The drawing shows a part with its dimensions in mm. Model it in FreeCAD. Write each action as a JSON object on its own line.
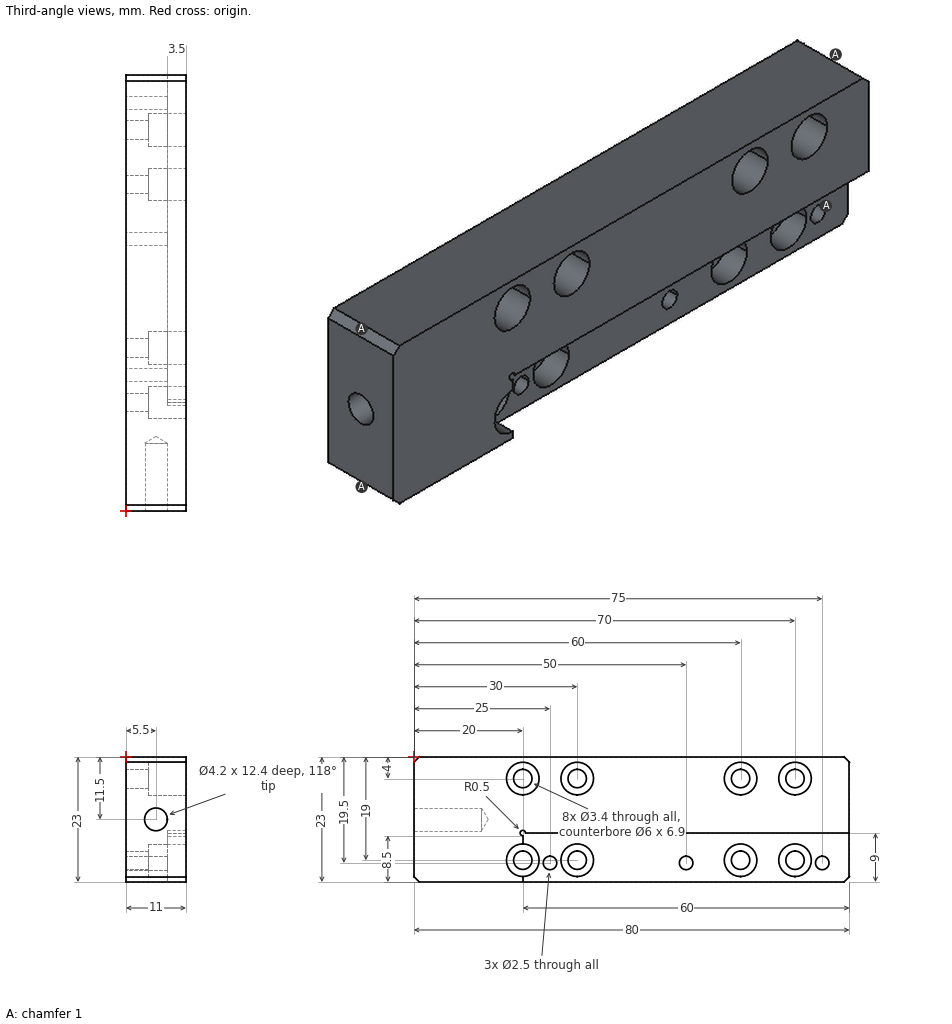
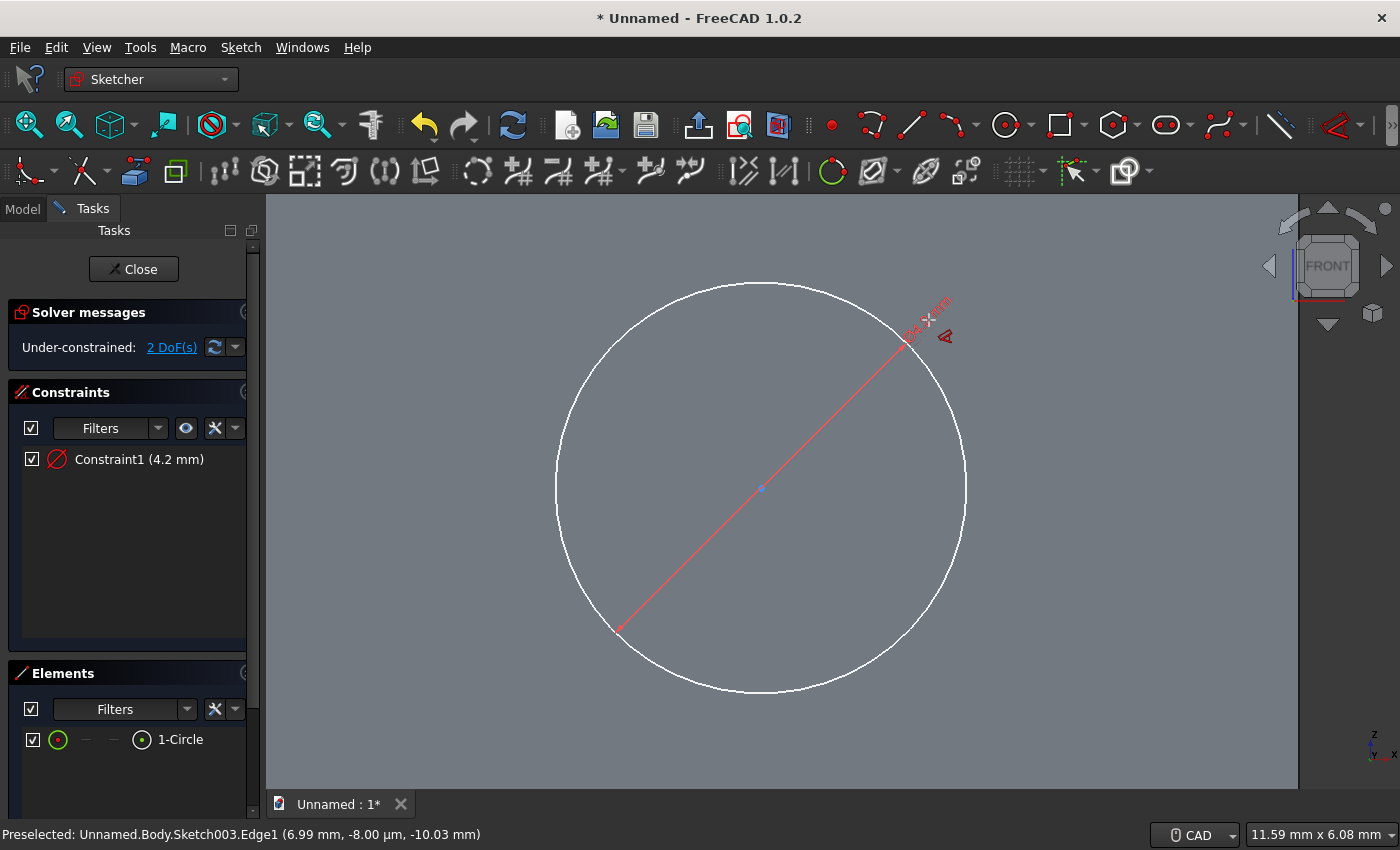
{"action": "left_click", "coordinate": [761, 488]}
{"action": "left_click", "coordinate": [528, 522]}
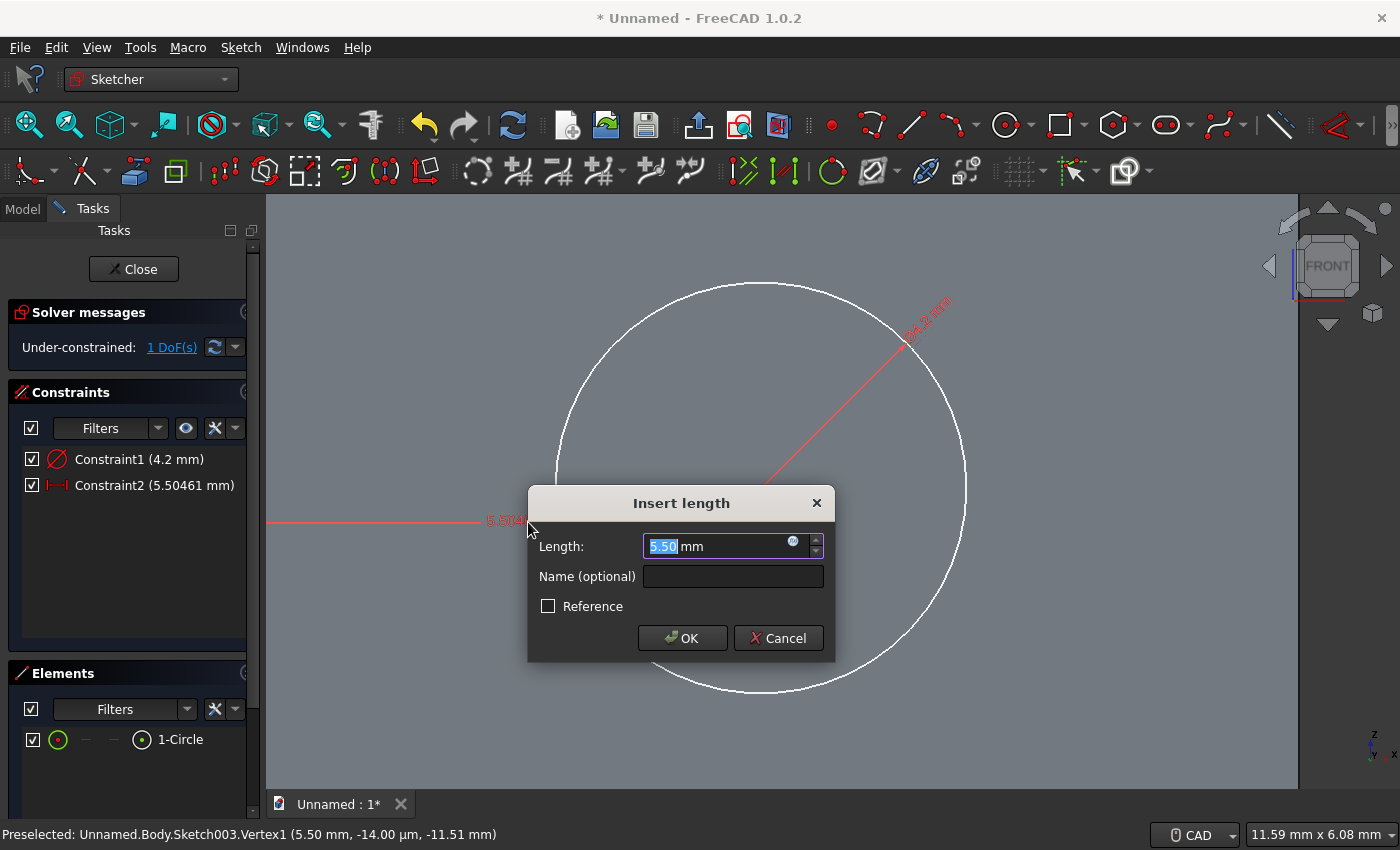
{"action": "type", "text": "5.5"}
{"action": "key", "text": "Return"}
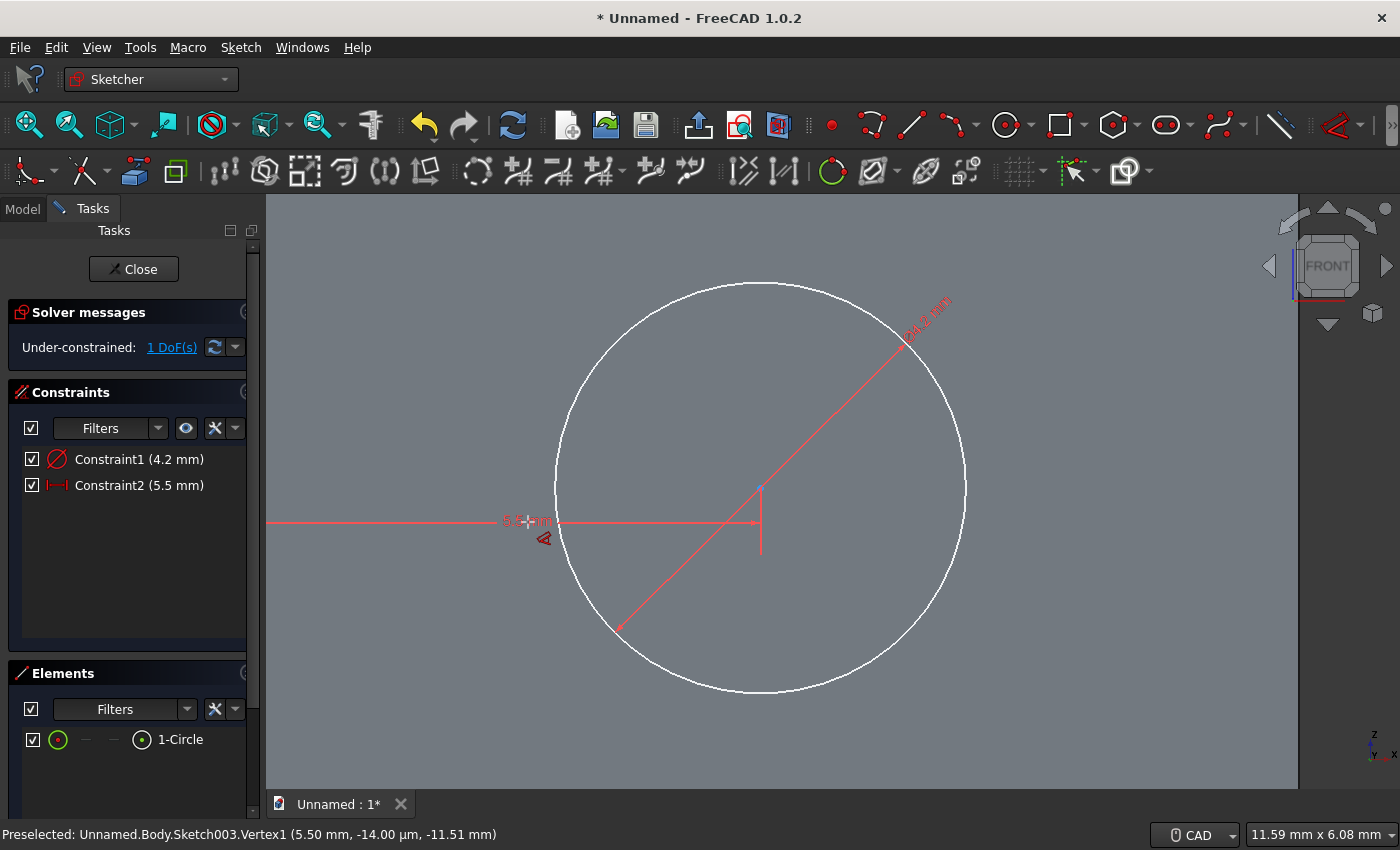
{"action": "left_click", "coordinate": [761, 488]}
{"action": "left_click", "coordinate": [795, 355]}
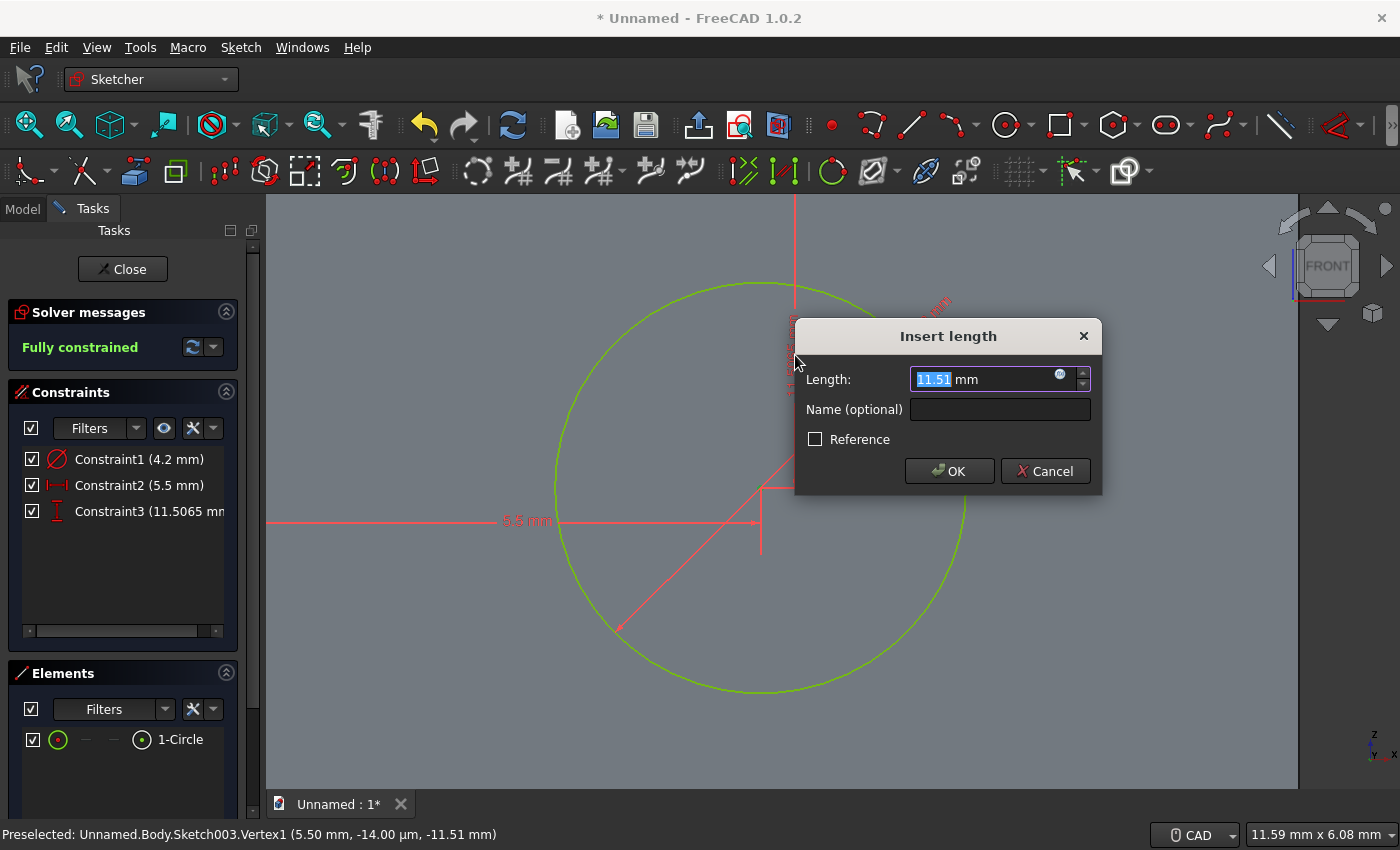
{"action": "type", "text": "11.5"}
{"action": "key", "text": "Return"}
{"action": "key", "text": "Escape"}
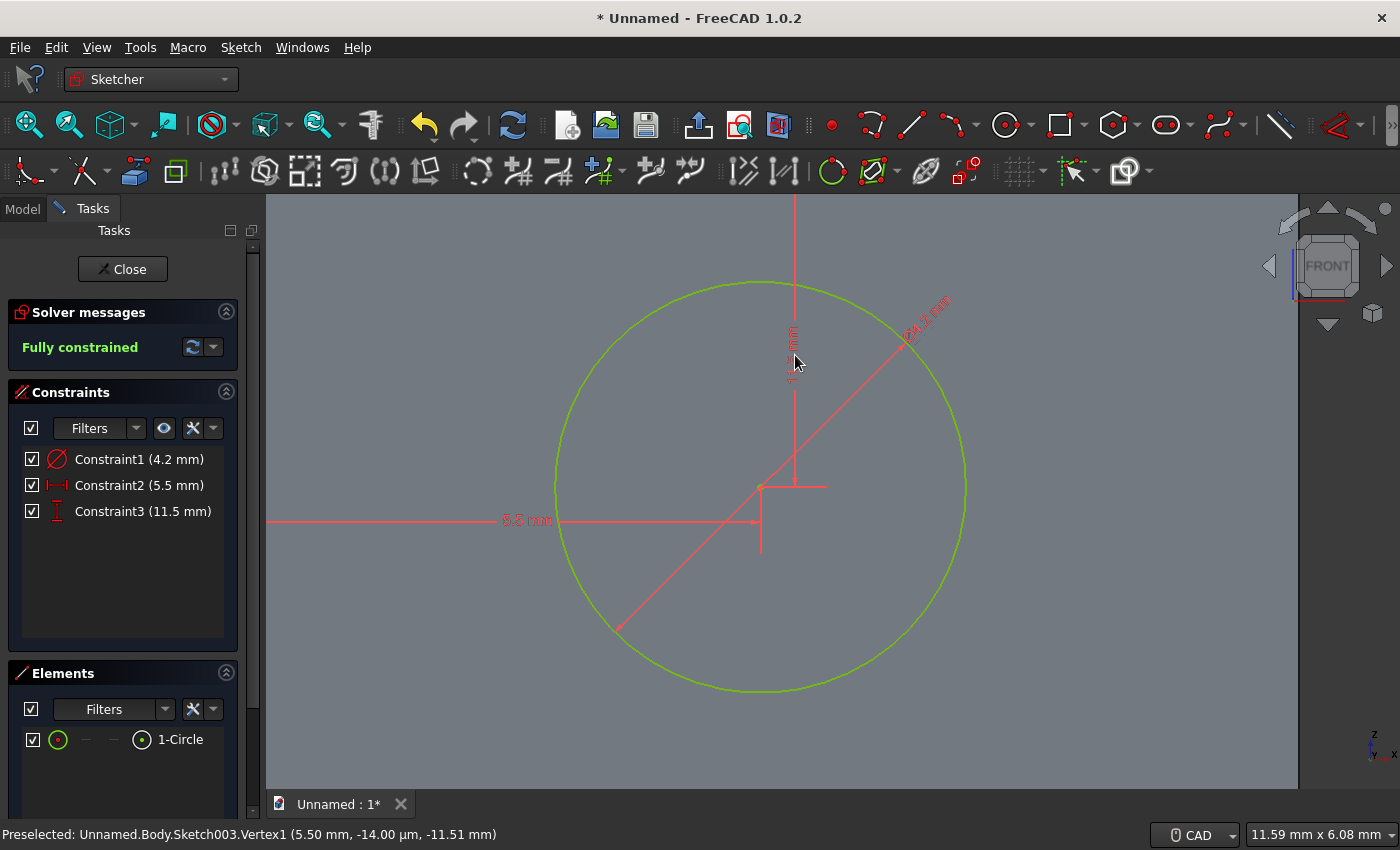
{"action": "left_click", "coordinate": [123, 269]}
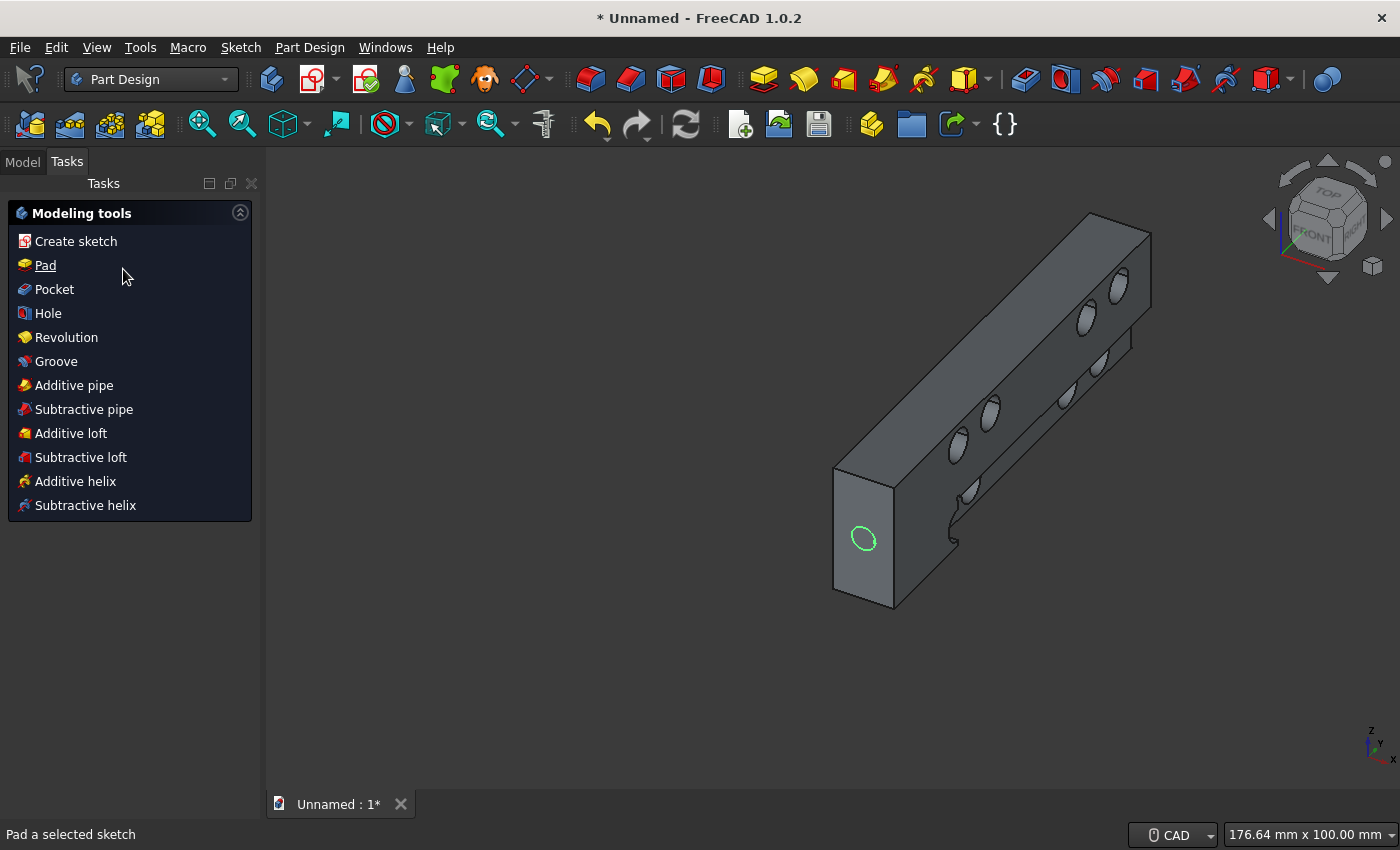
{"action": "left_click", "coordinate": [1066, 80]}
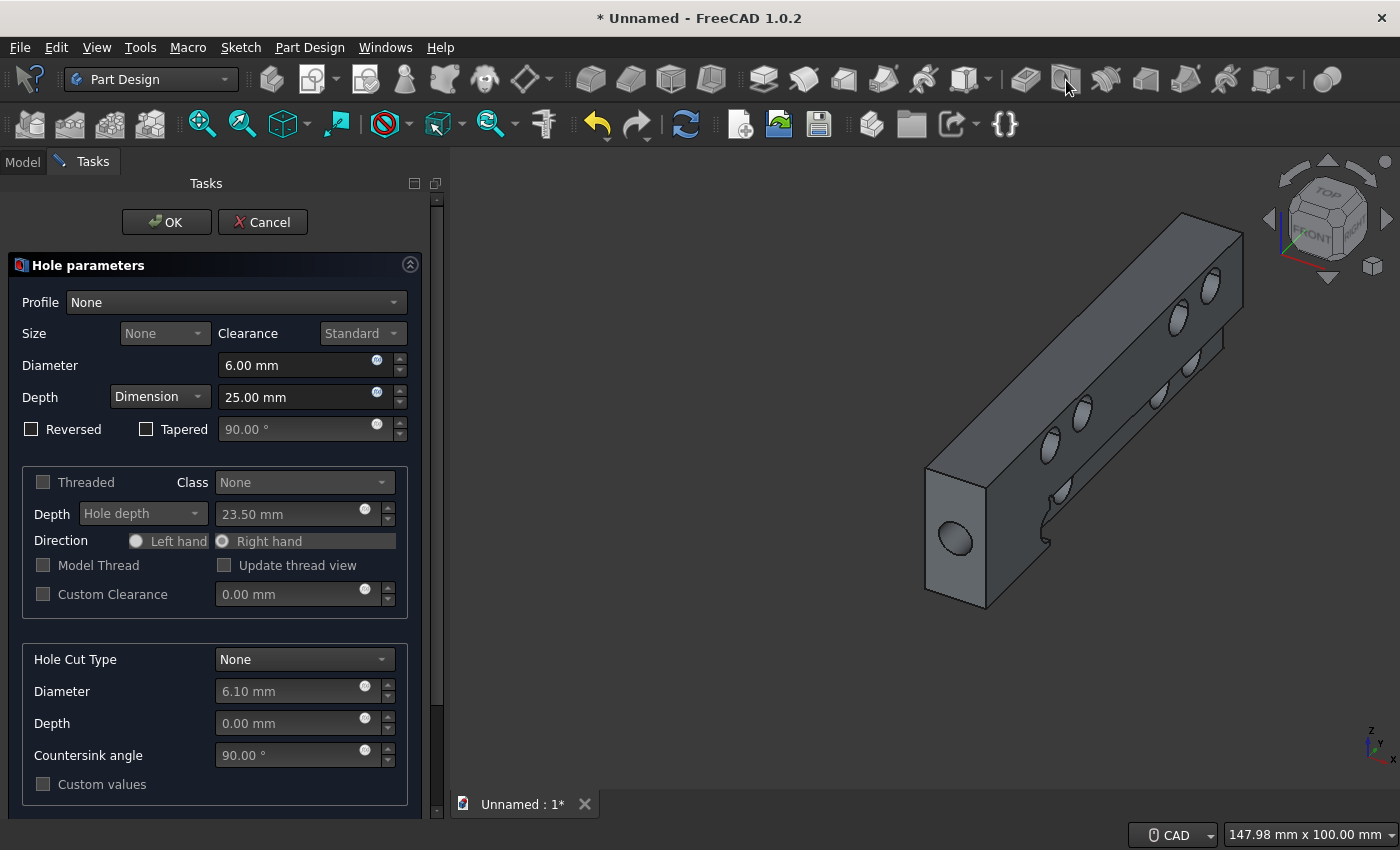
{"action": "triple_click", "coordinate": [305, 365]}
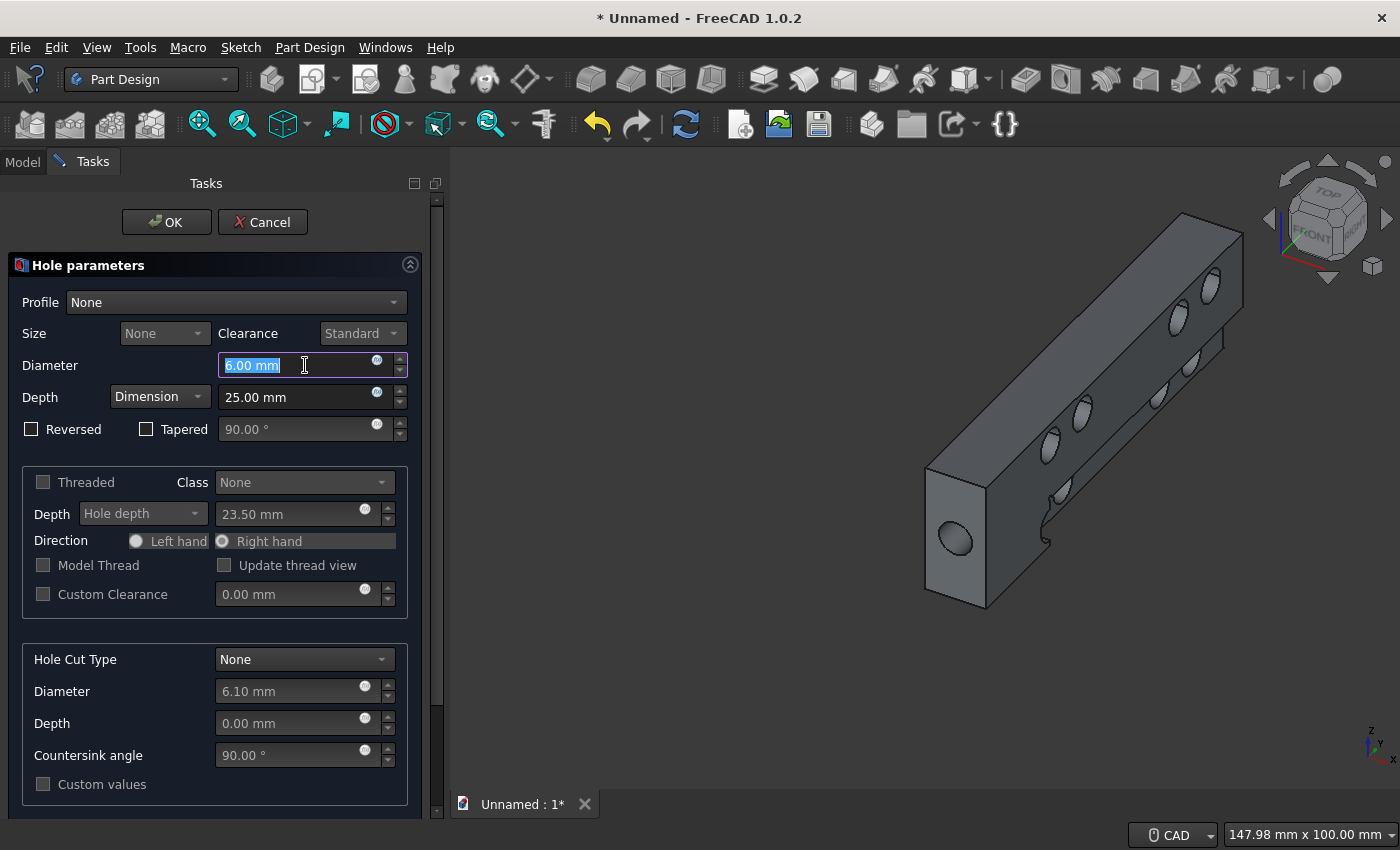
{"action": "type", "text": "4.2"}
{"action": "key", "text": "Tab"}